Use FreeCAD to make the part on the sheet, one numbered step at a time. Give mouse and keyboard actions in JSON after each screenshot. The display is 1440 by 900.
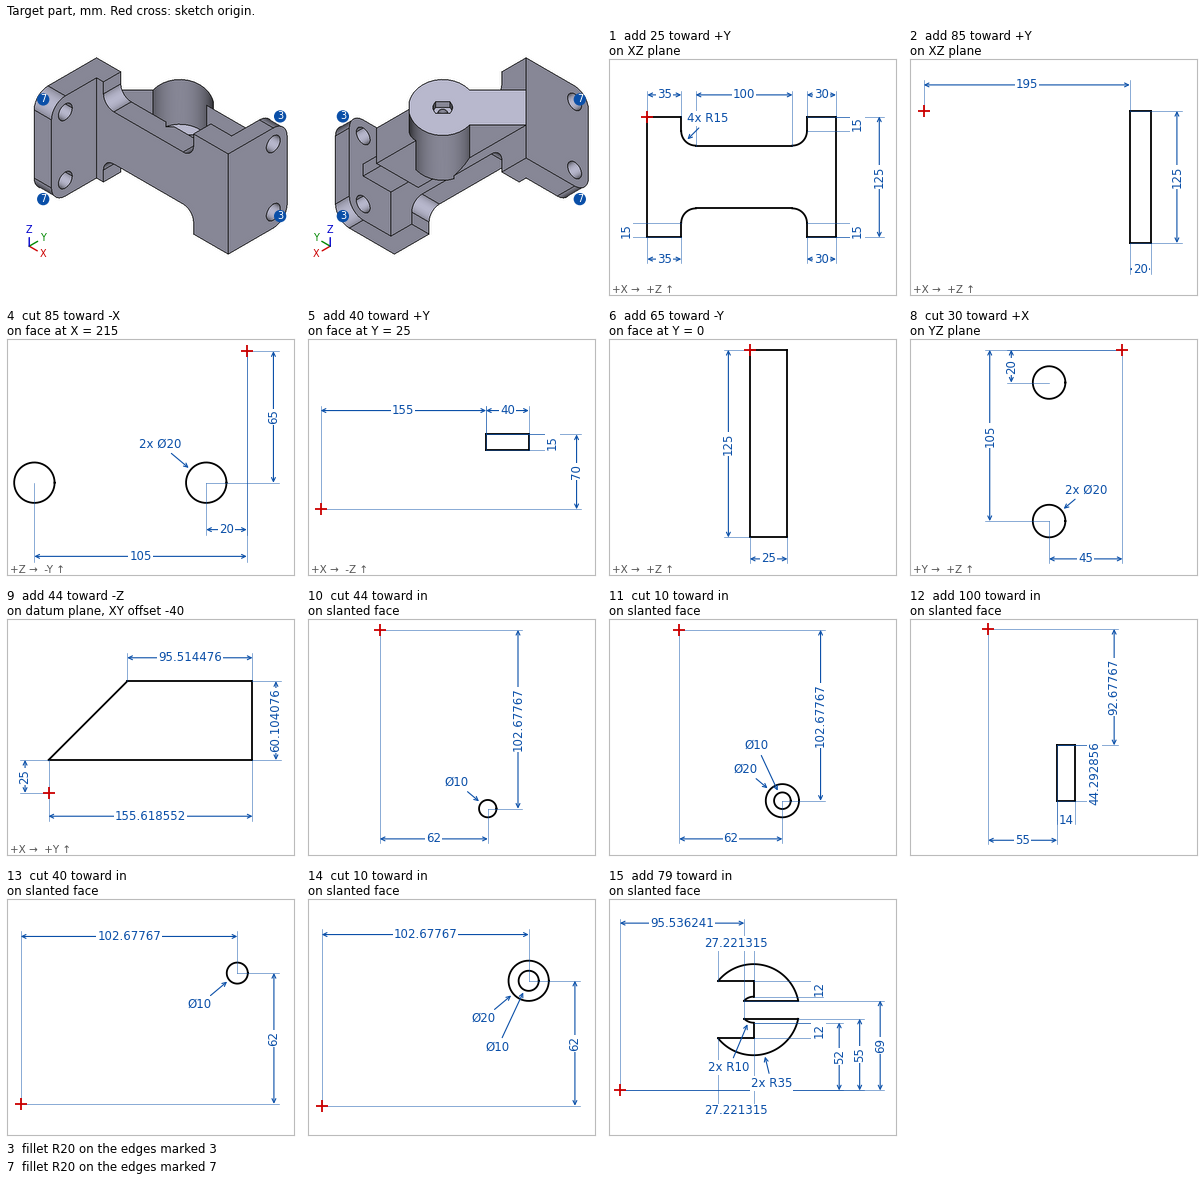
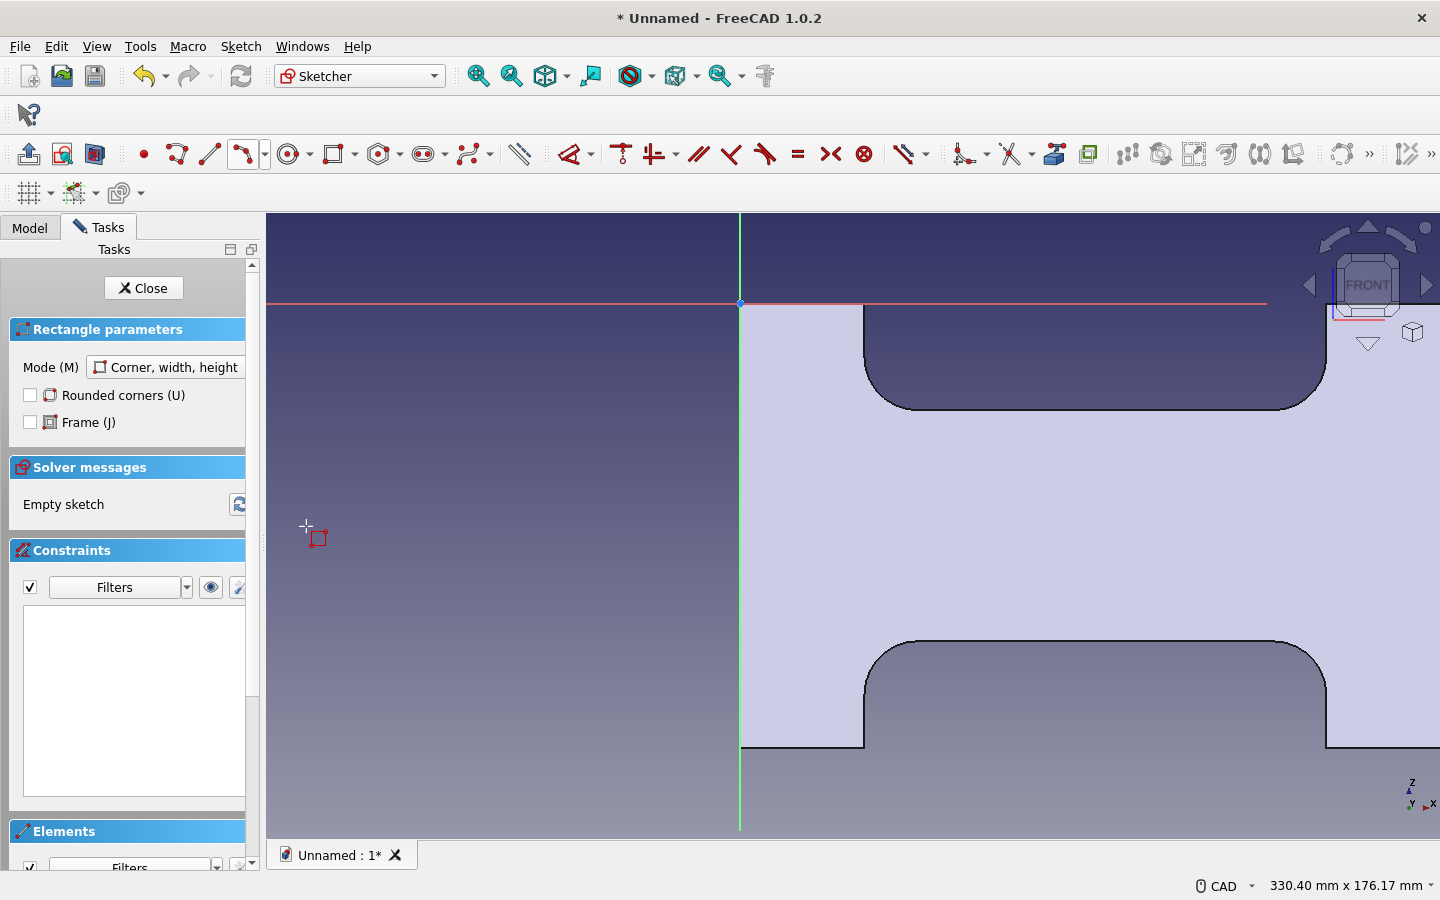
{"action": "left_click", "coordinate": [740, 304]}
{"action": "left_click", "coordinate": [829, 748]}
{"action": "key", "text": "Escape"}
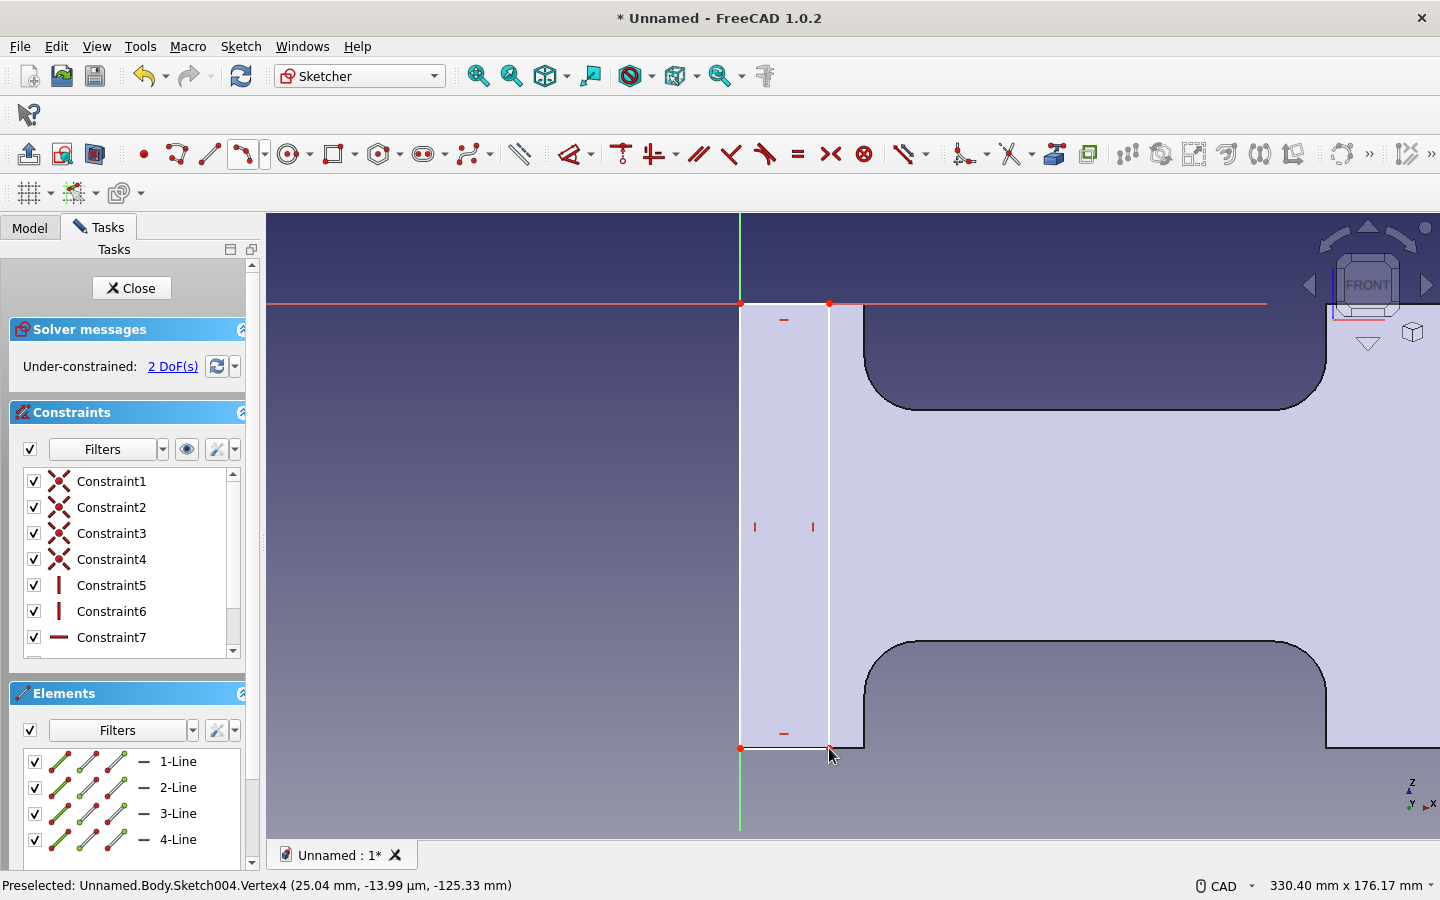
{"action": "left_click", "coordinate": [568, 154]}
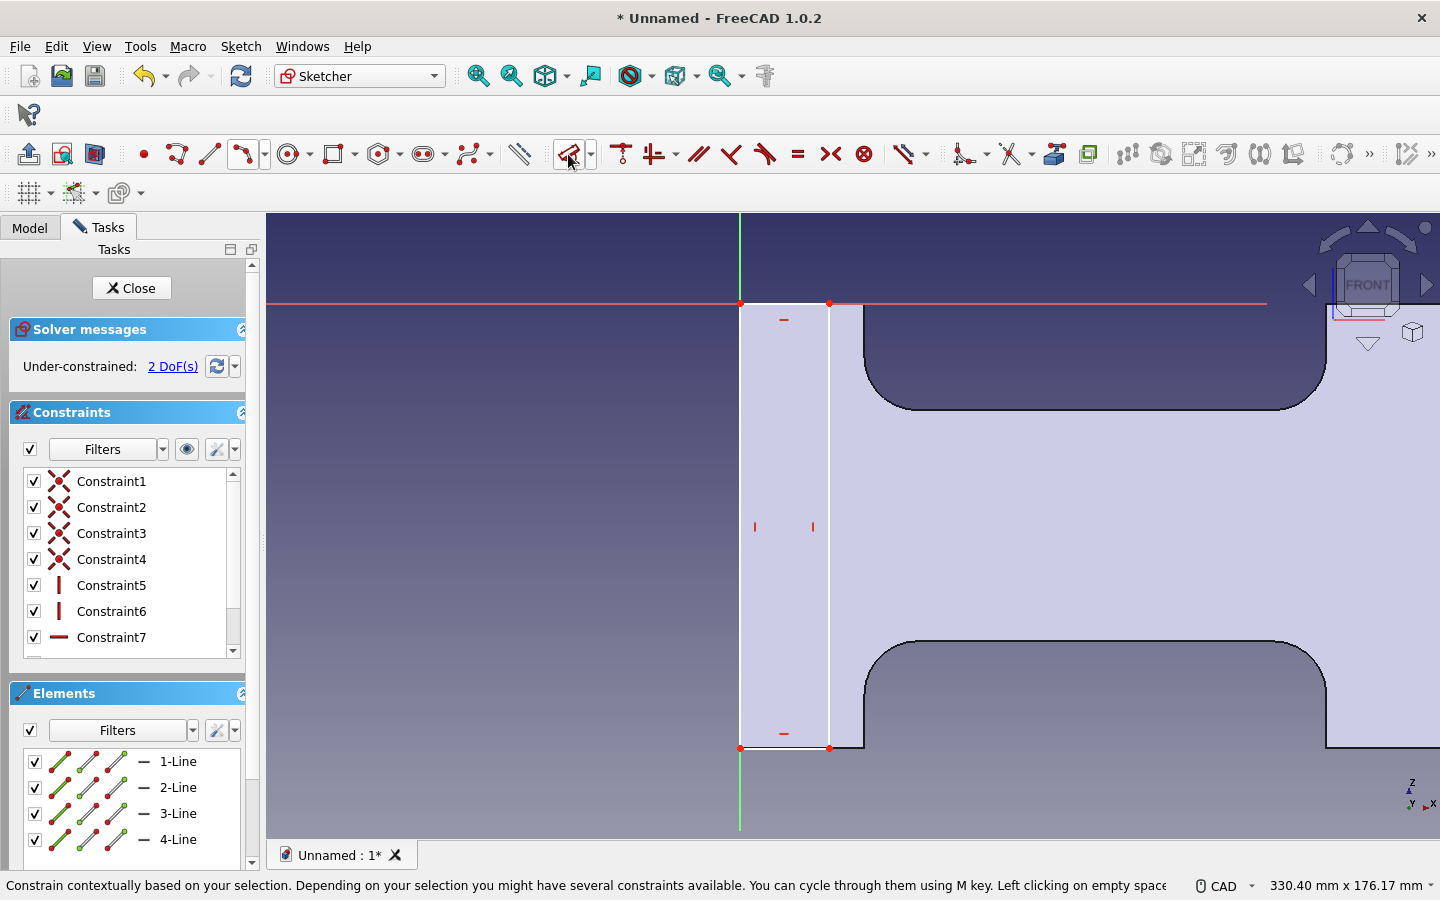
{"action": "left_click", "coordinate": [767, 749]}
{"action": "left_click", "coordinate": [785, 783]}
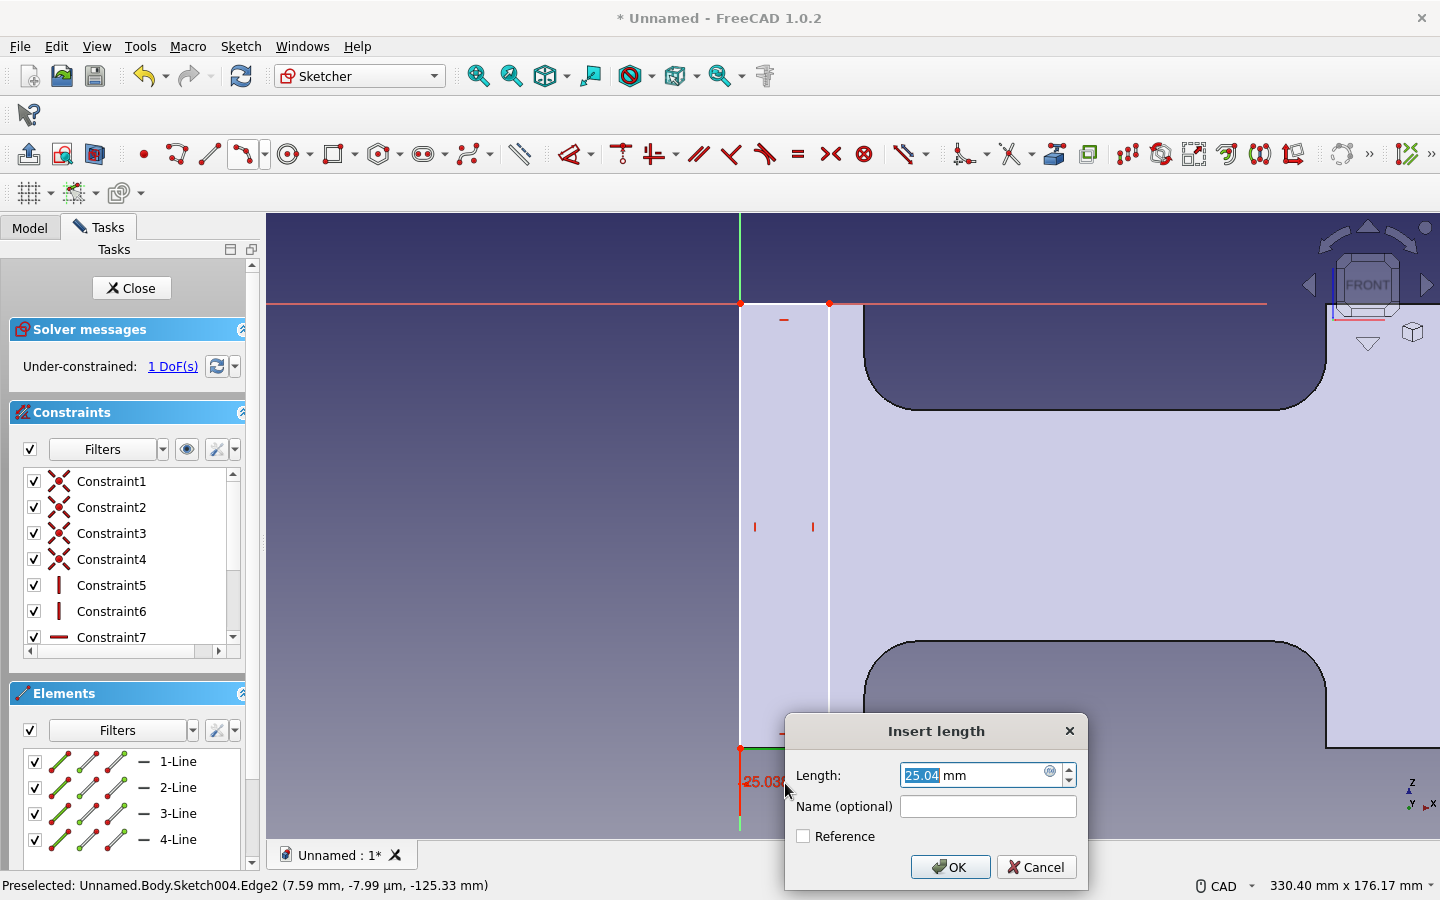
{"action": "type", "text": "25"}
{"action": "key", "text": "Return"}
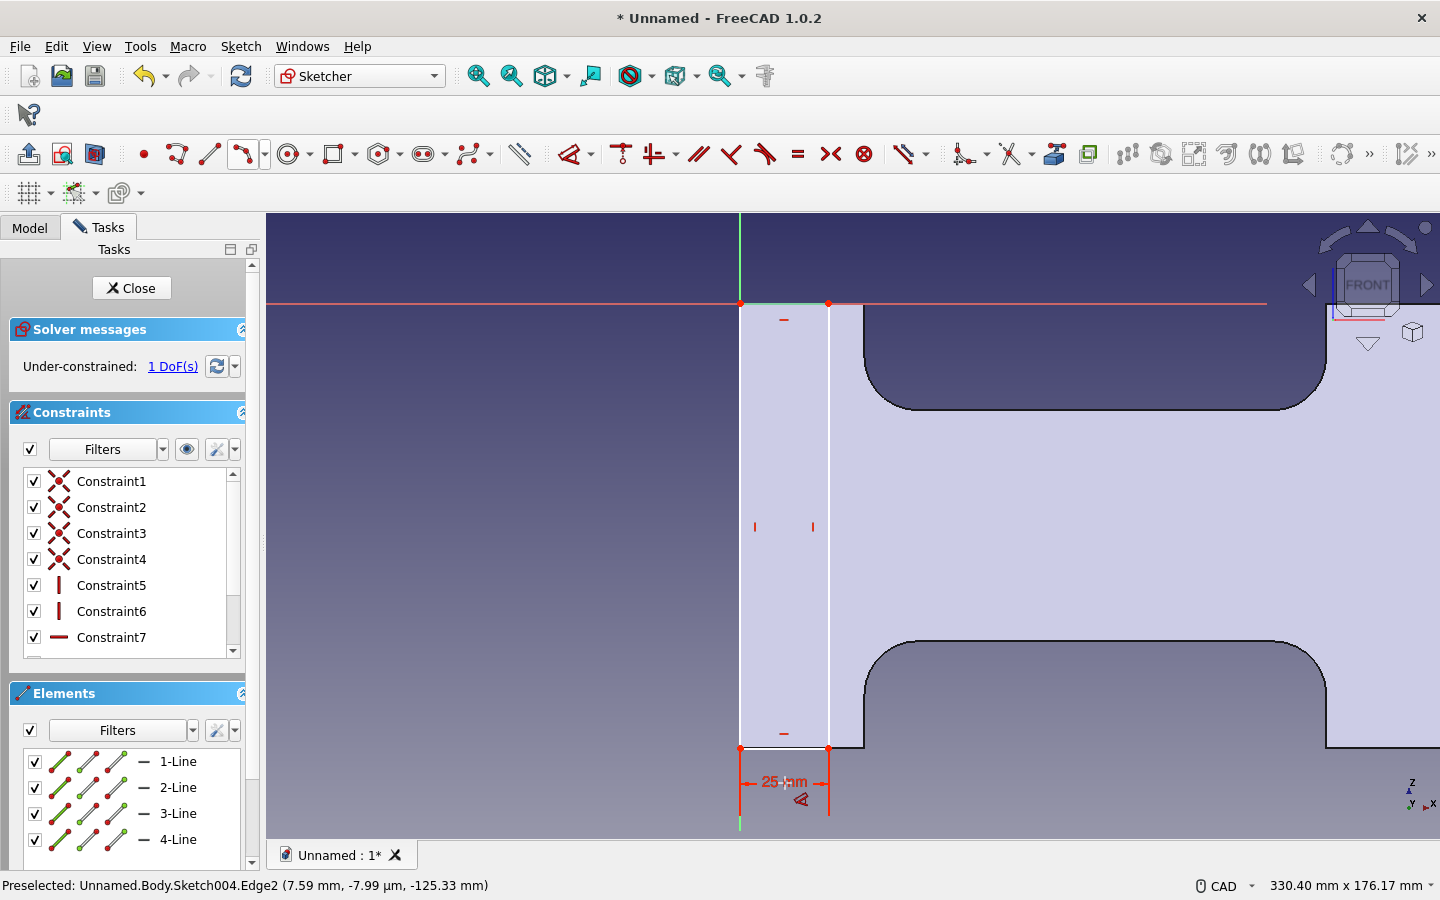
{"action": "left_click", "coordinate": [740, 437]}
{"action": "left_click", "coordinate": [706, 526]}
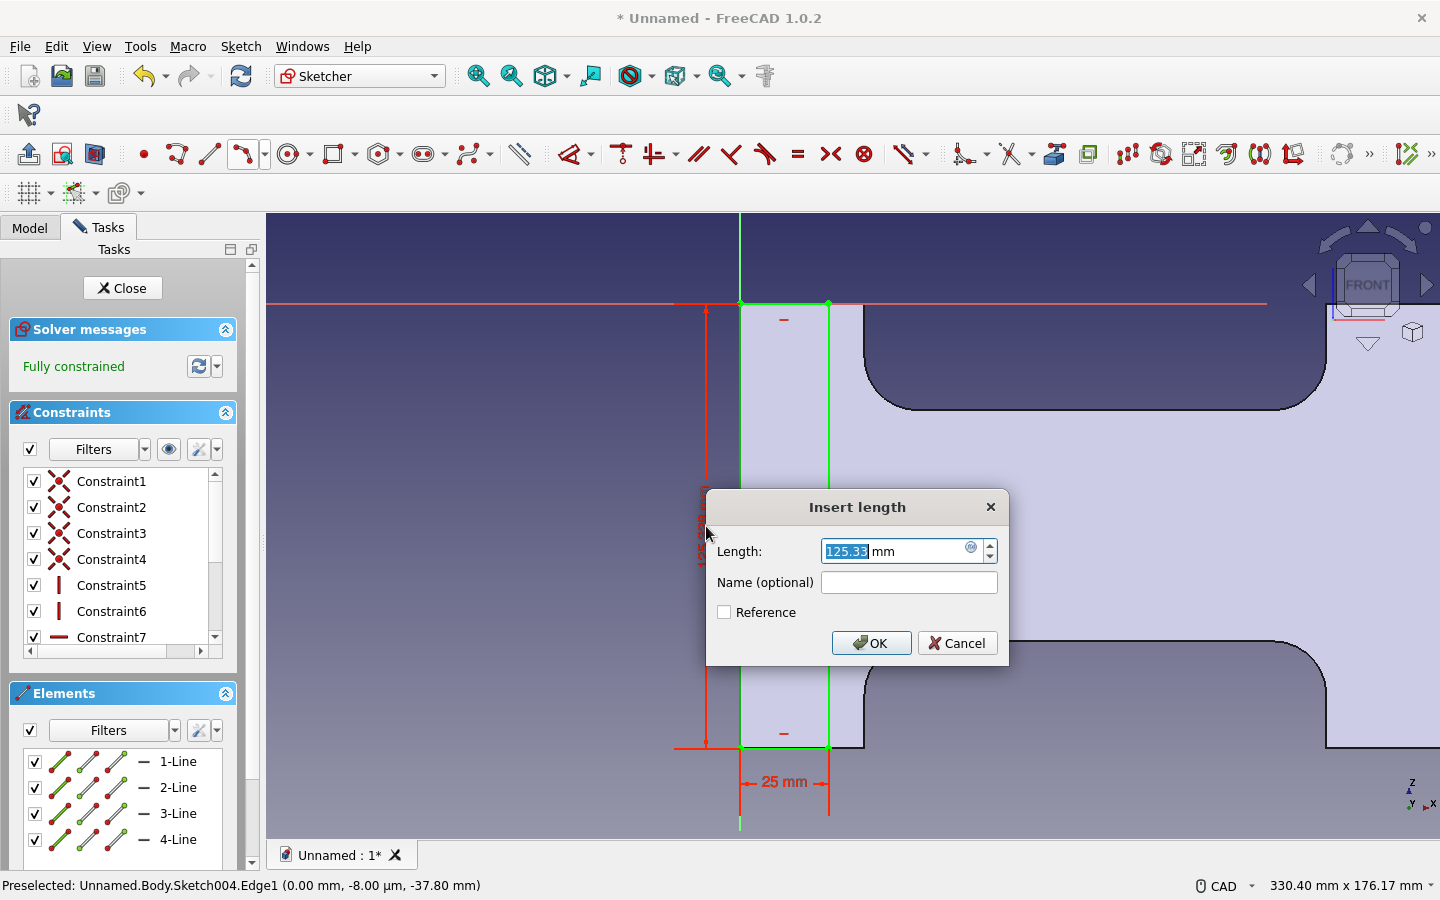
{"action": "type", "text": "125"}
{"action": "key", "text": "Return"}
{"action": "key", "text": "Escape"}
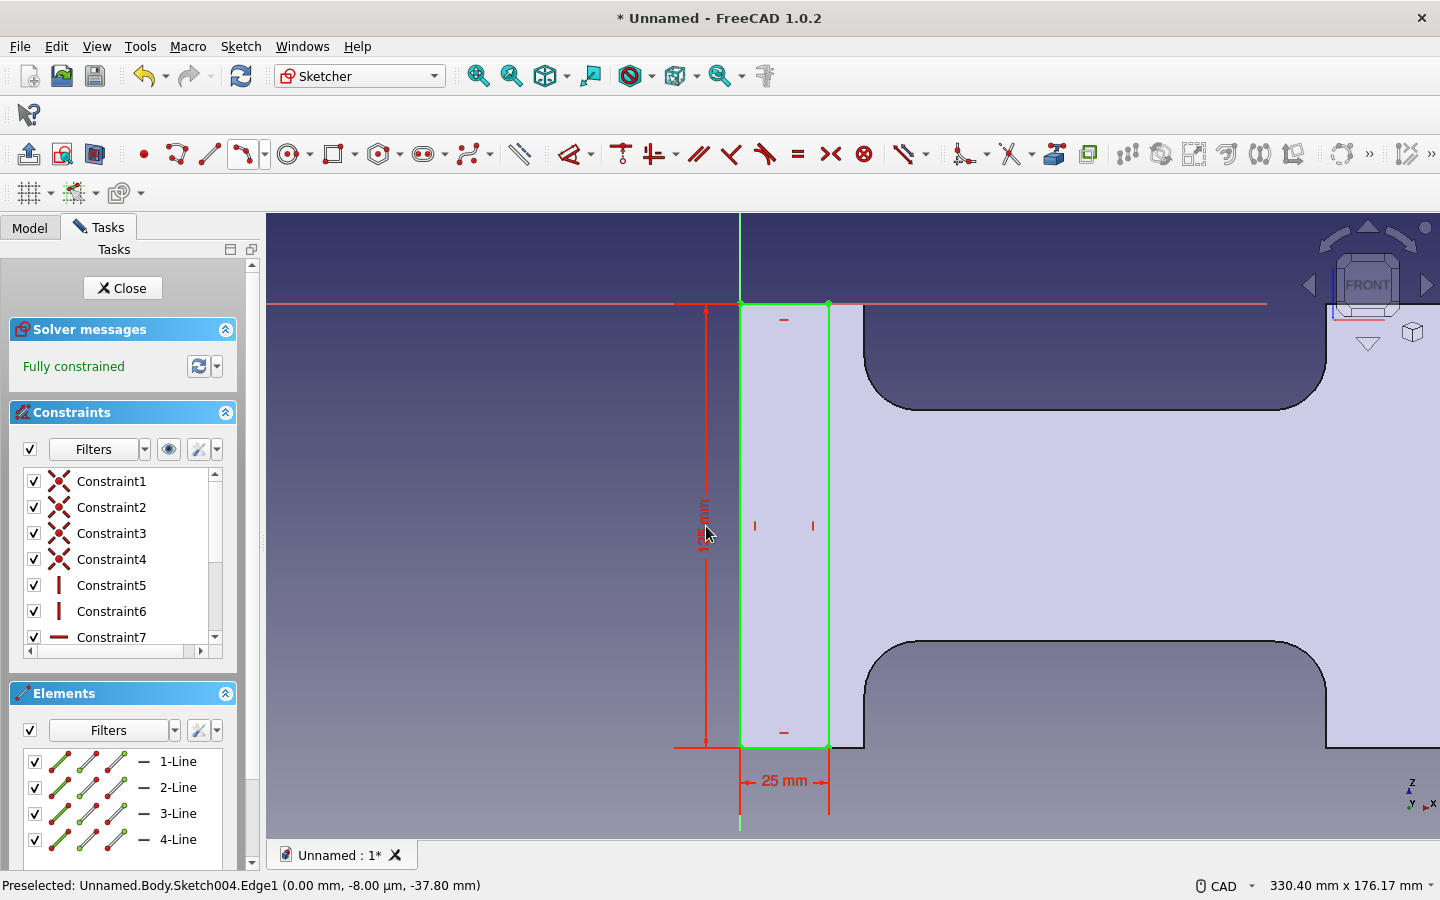
{"action": "left_click", "coordinate": [123, 288]}